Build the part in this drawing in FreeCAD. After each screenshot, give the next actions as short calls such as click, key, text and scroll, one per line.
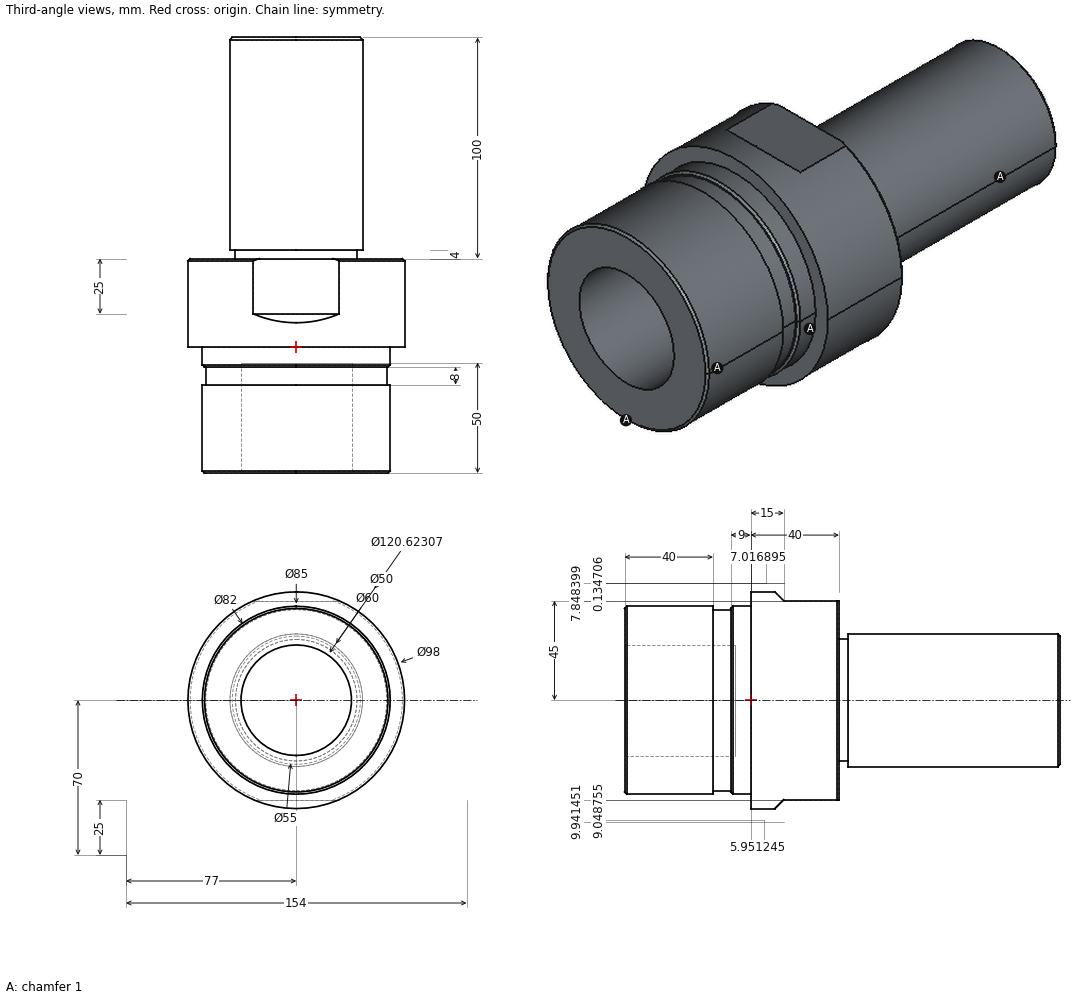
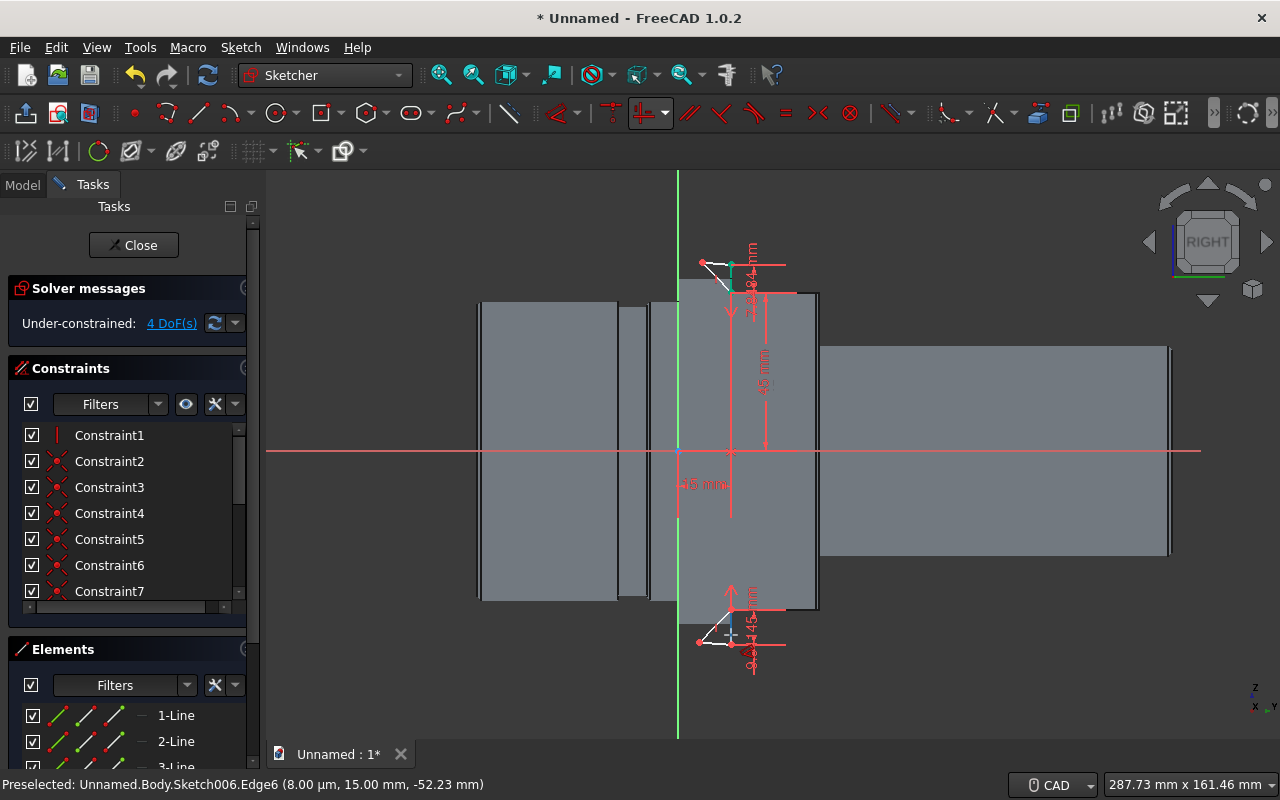
scroll(703, 263, up, 3)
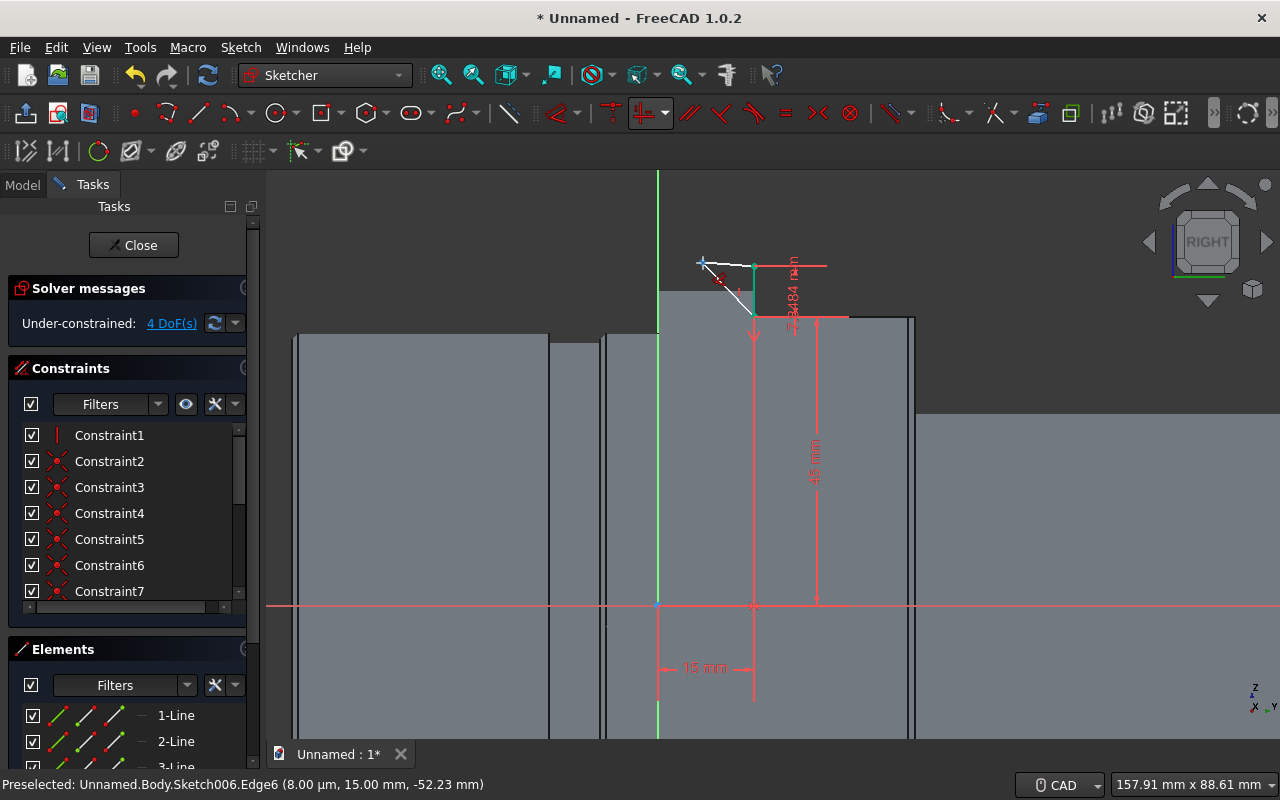
click(702, 262)
click(680, 228)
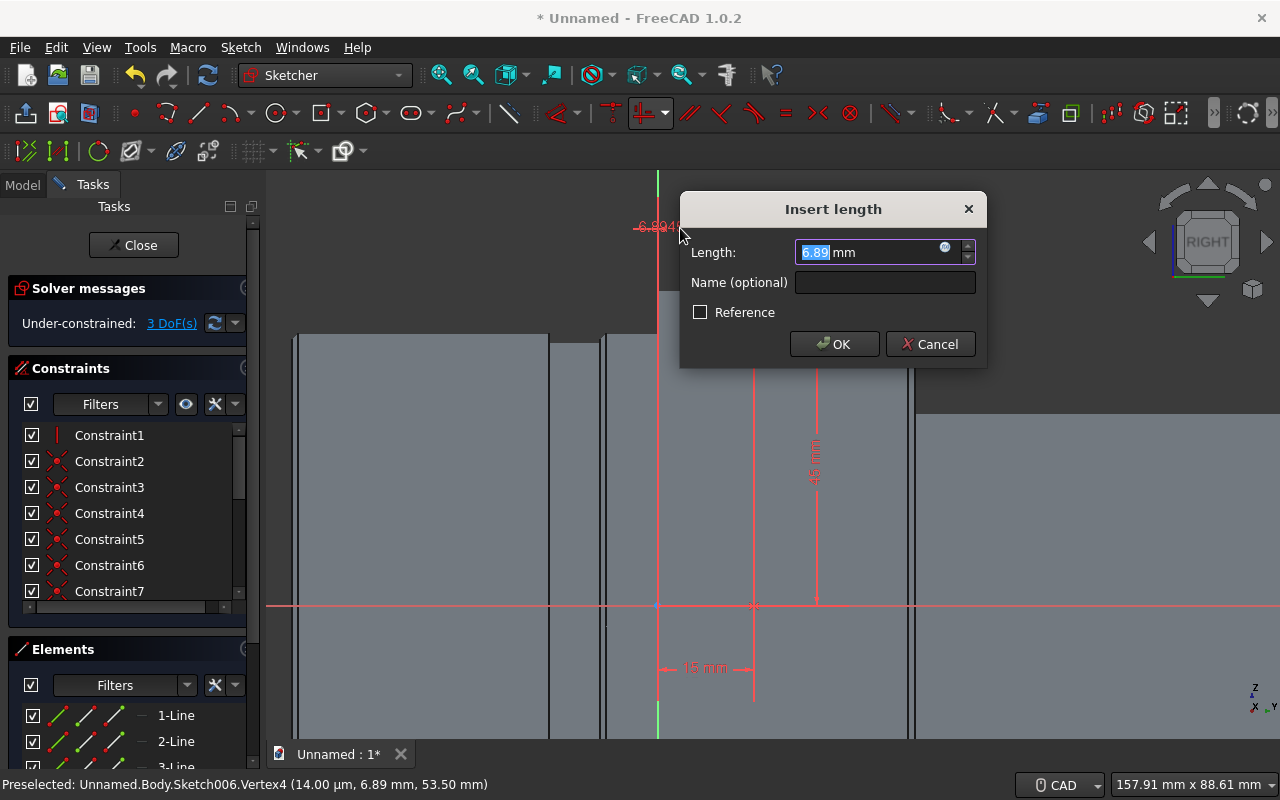
text(7.016895)
key(Return)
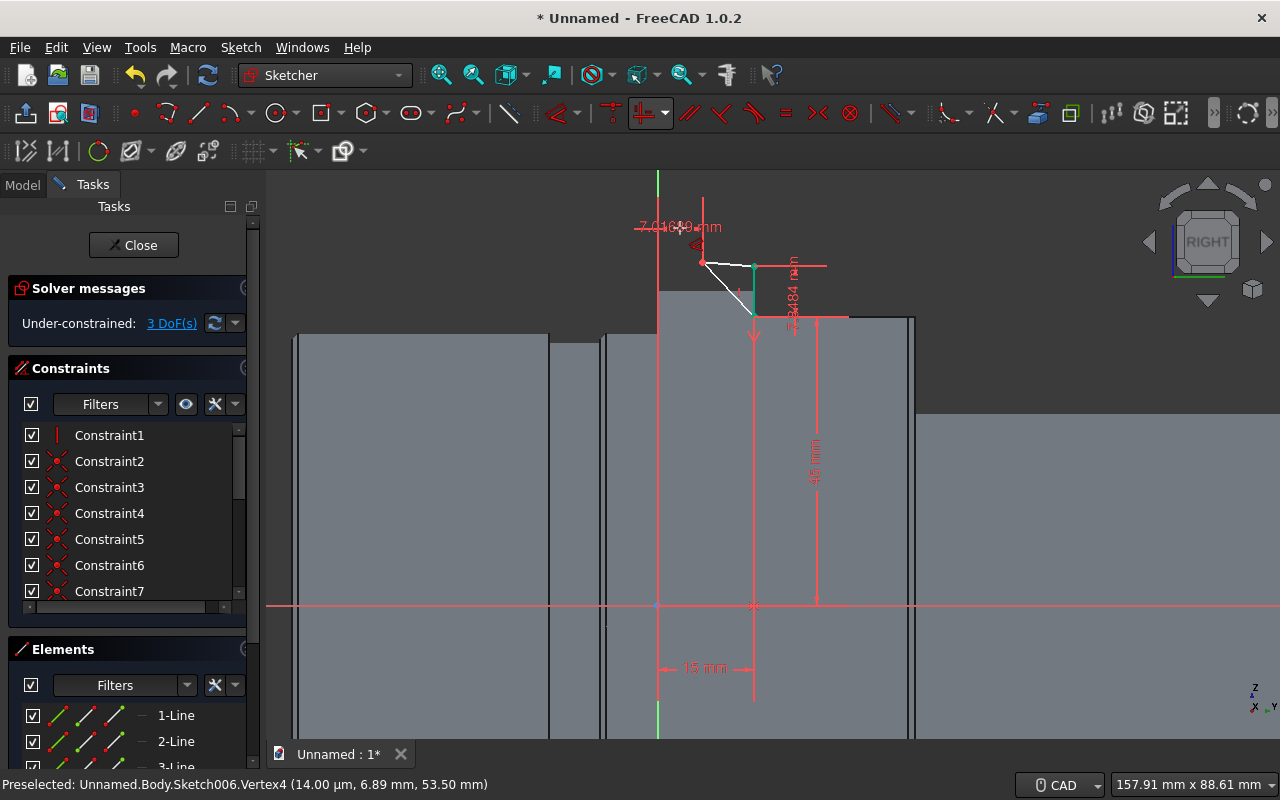
scroll(703, 263, down, 3)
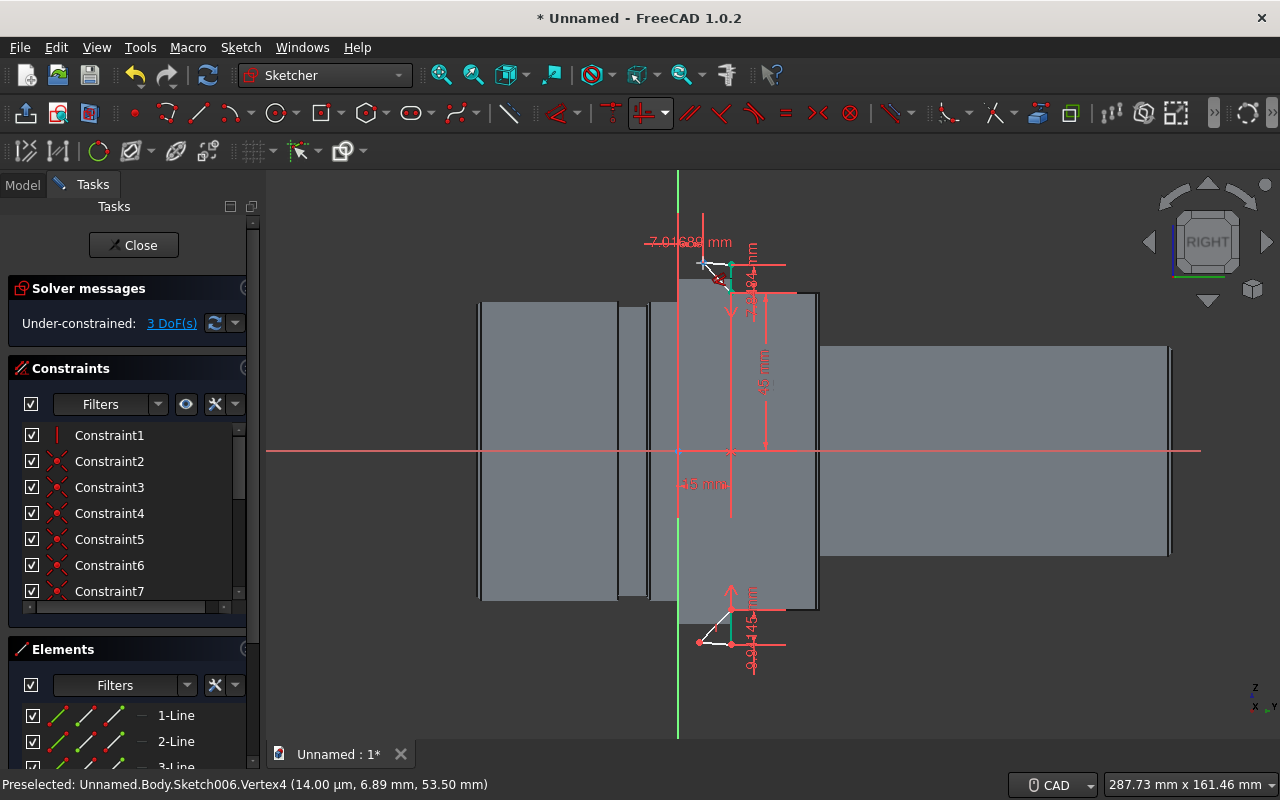
scroll(700, 643, up, 4)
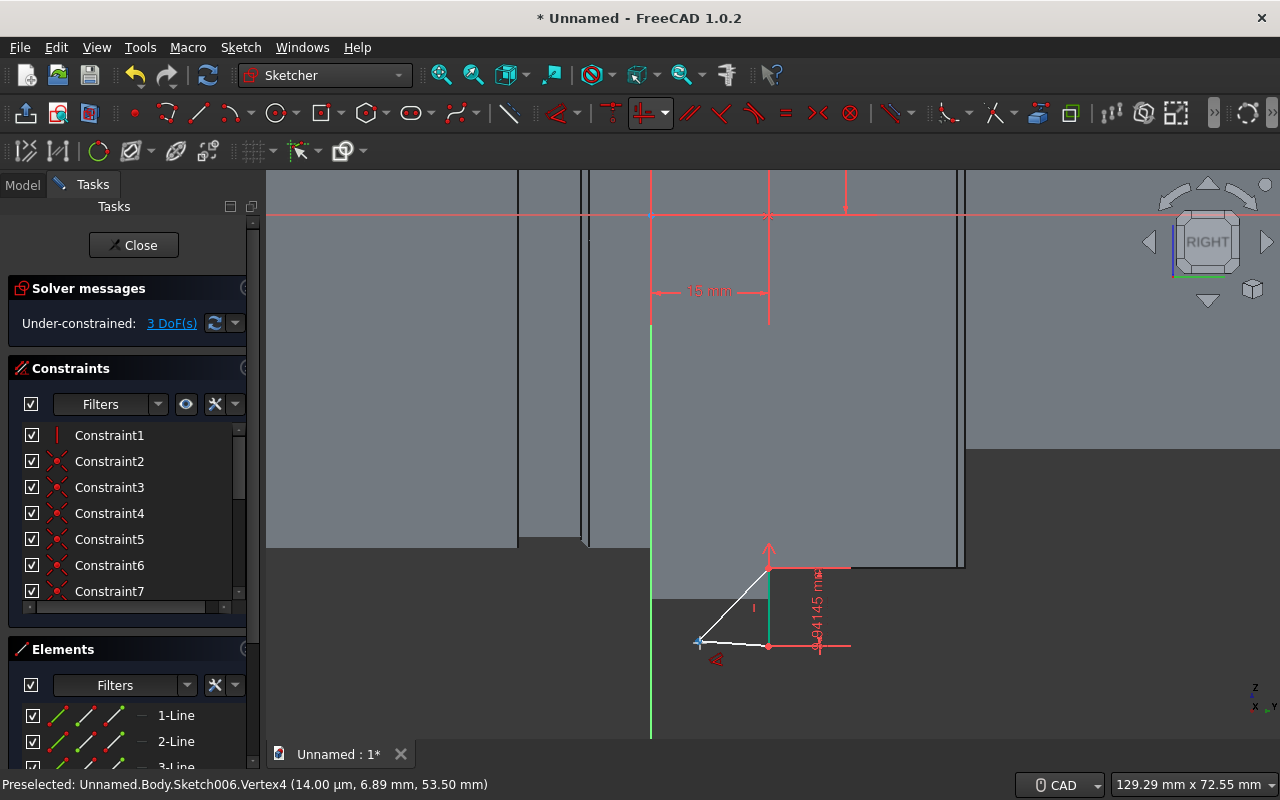
click(699, 641)
click(675, 675)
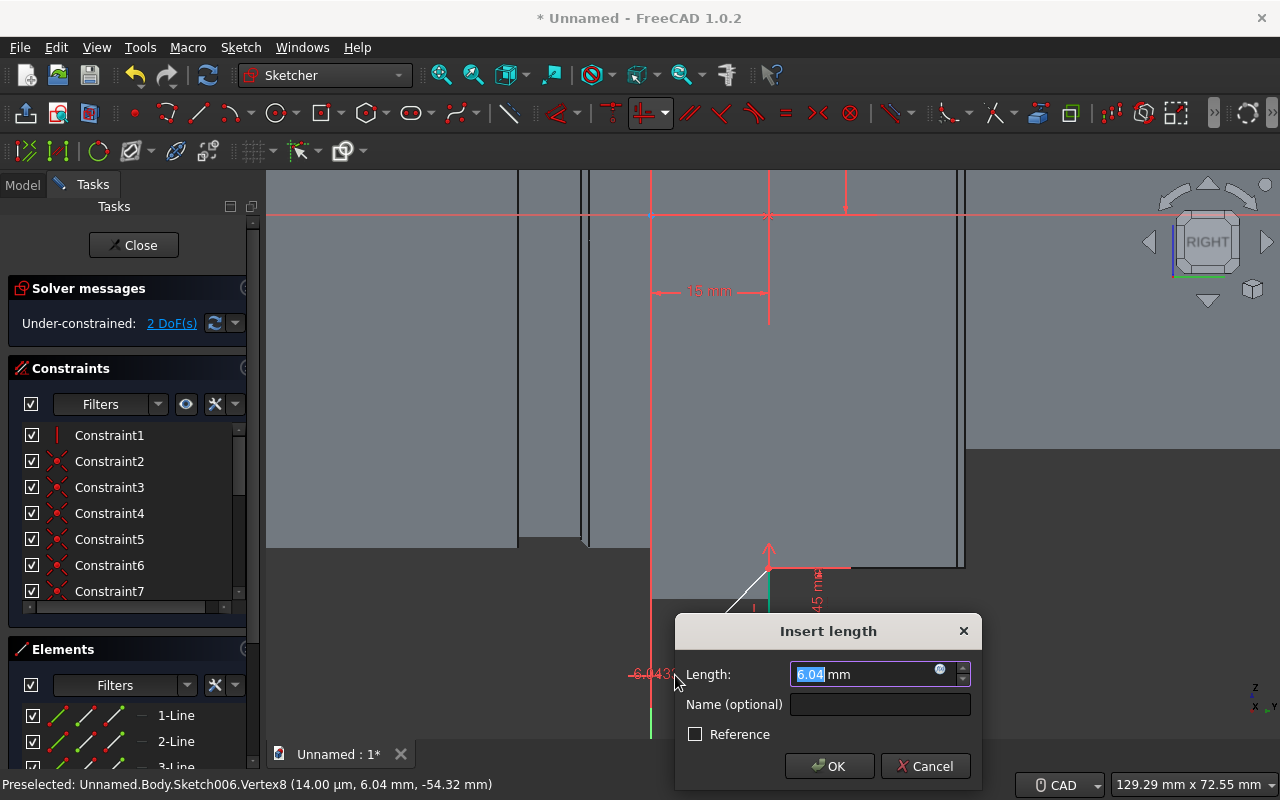
text(5.951245)
key(Return)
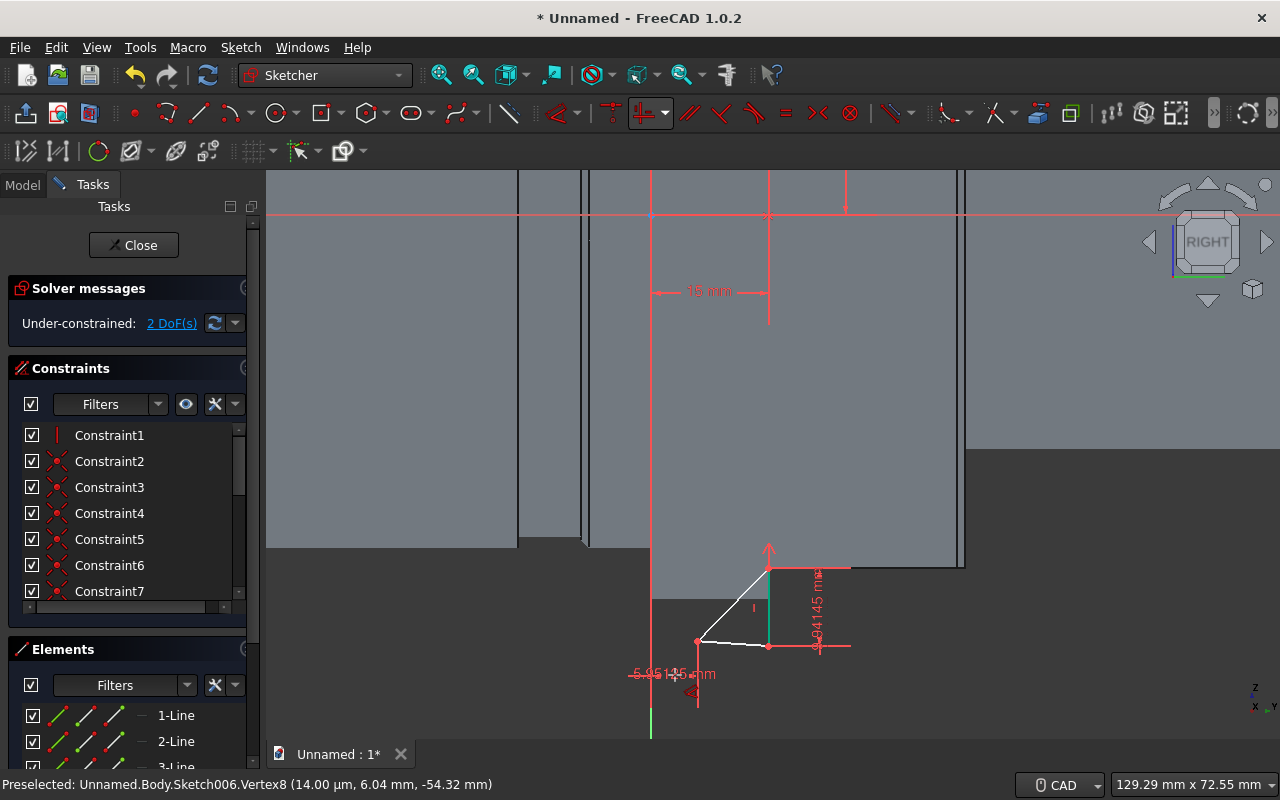
scroll(700, 644, down, 4)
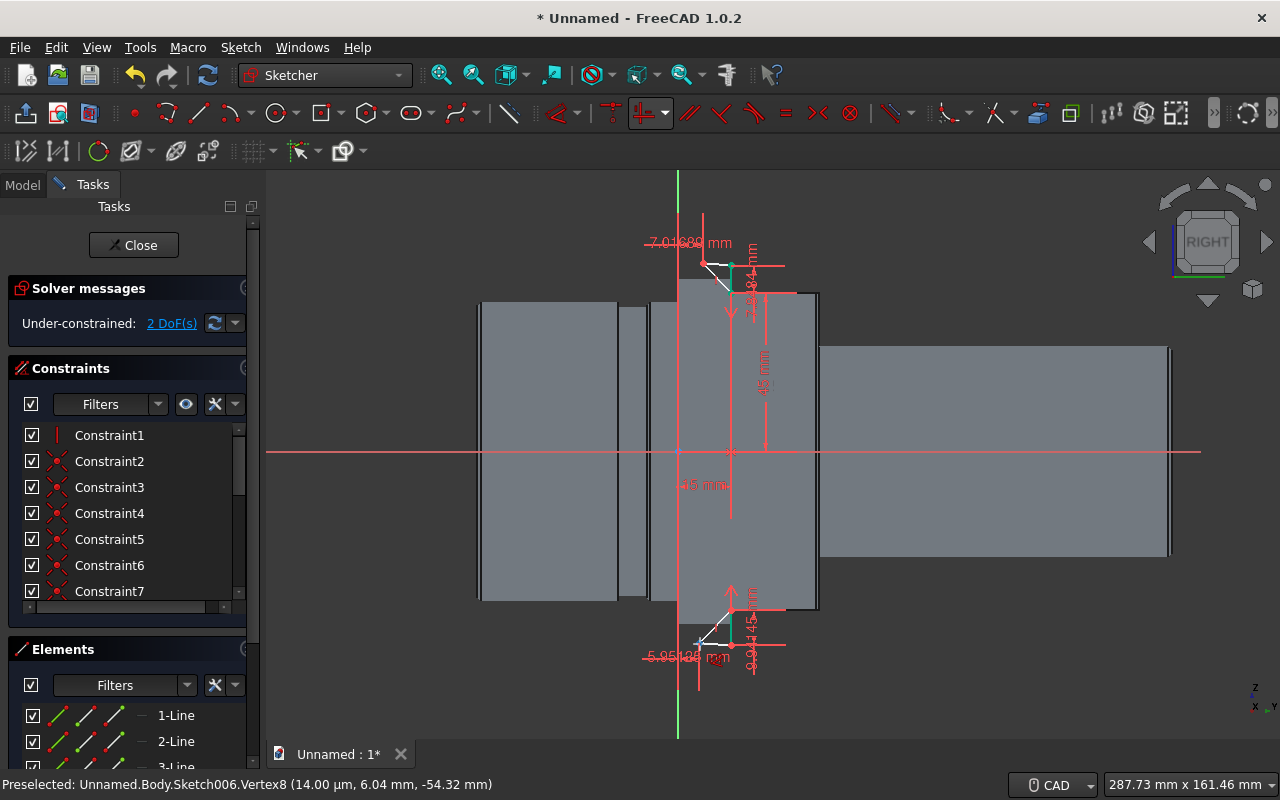
scroll(723, 265, up, 23)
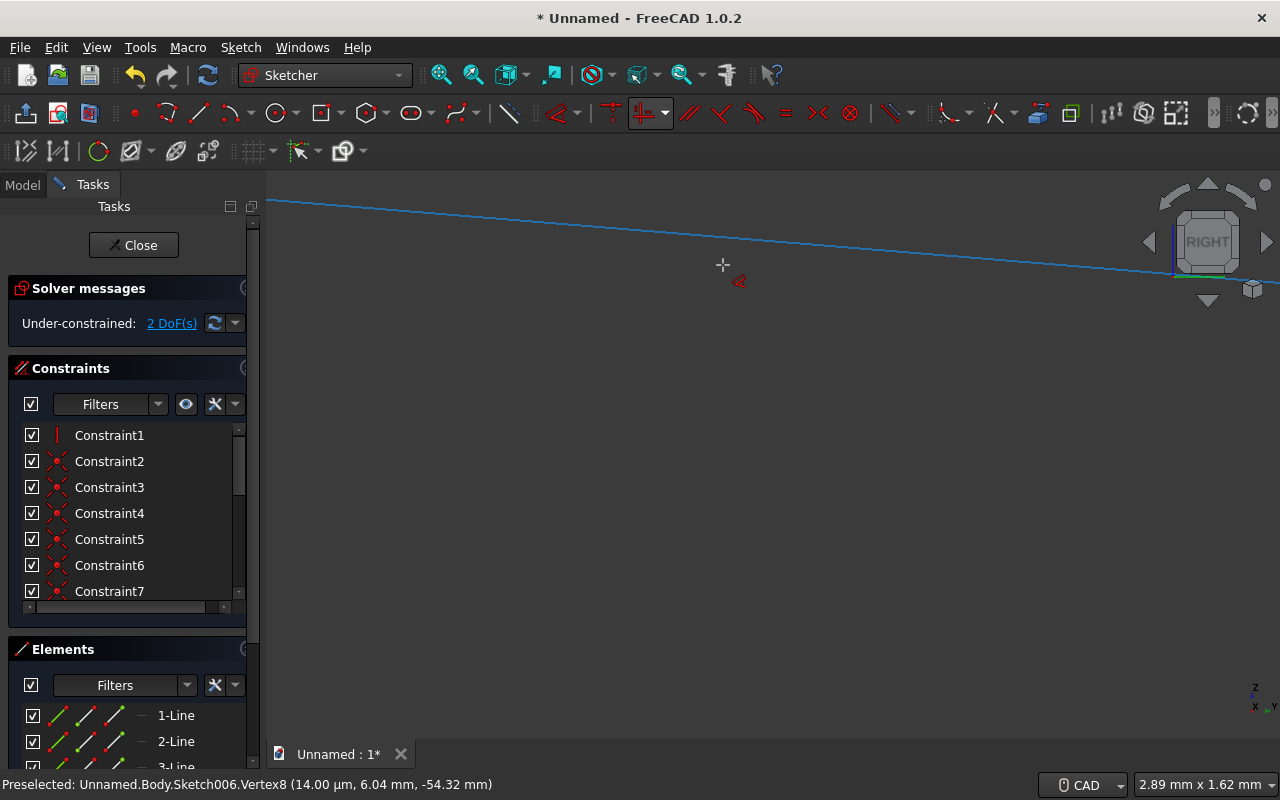
click(657, 232)